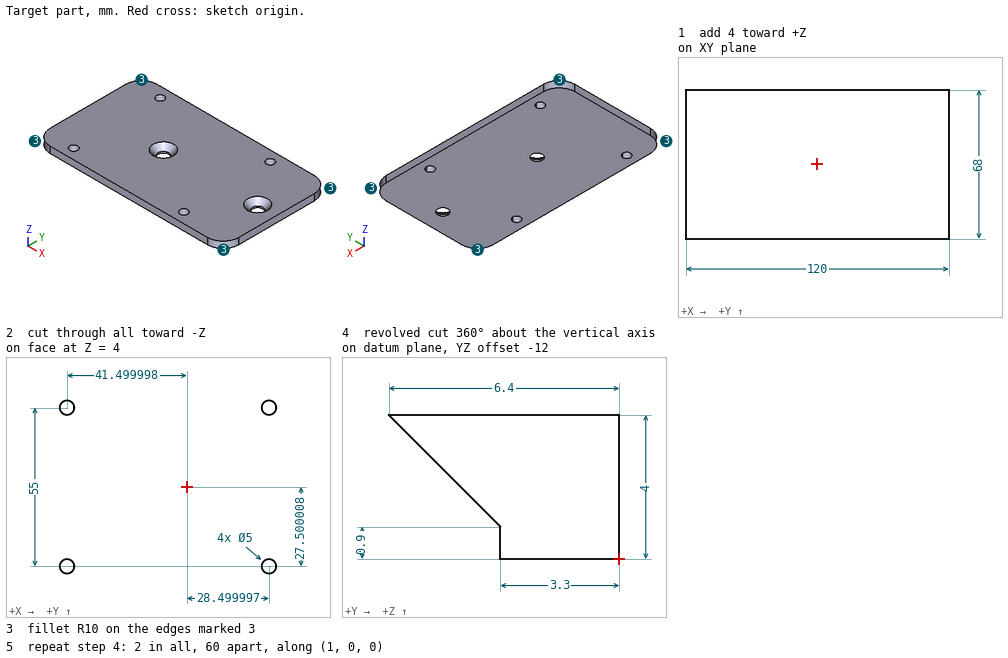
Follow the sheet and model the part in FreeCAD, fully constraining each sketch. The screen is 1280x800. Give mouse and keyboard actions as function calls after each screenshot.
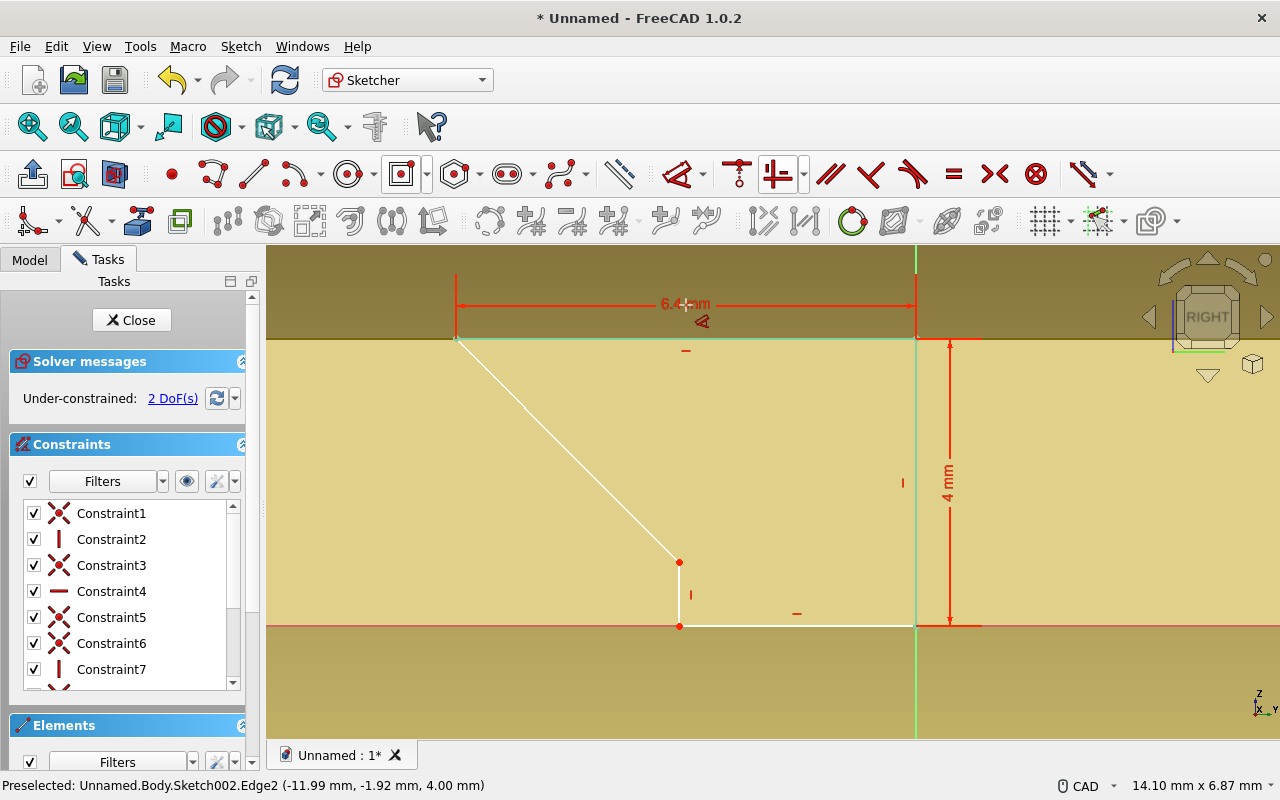
click(679, 582)
click(645, 595)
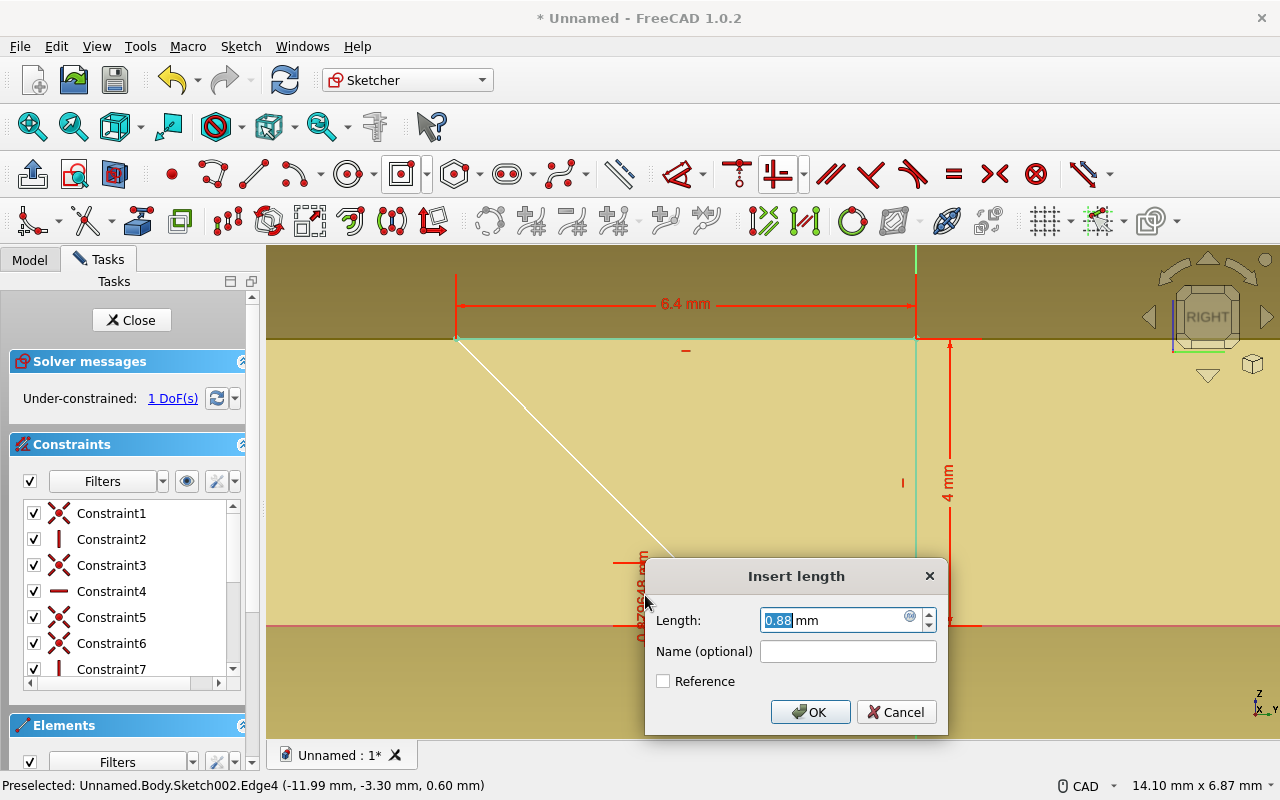
text(0.9)
key(Return)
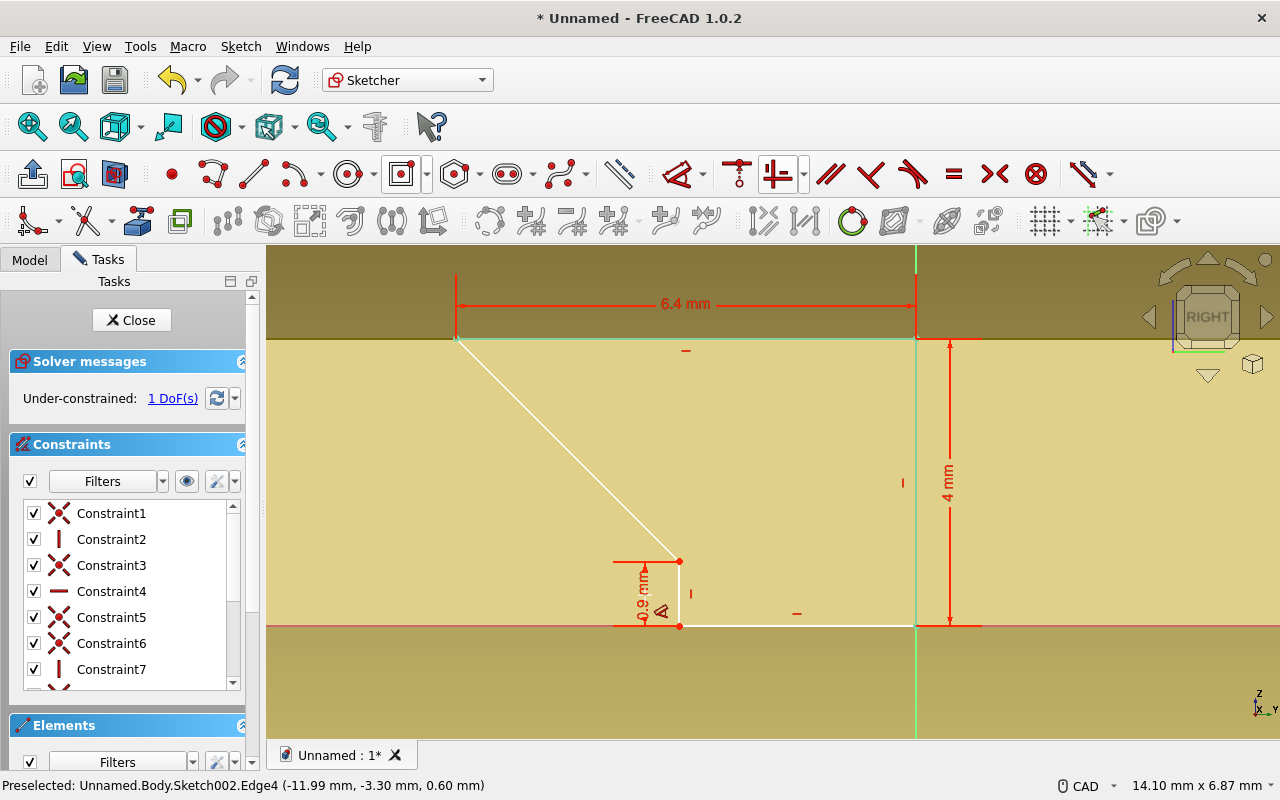
click(750, 626)
click(798, 660)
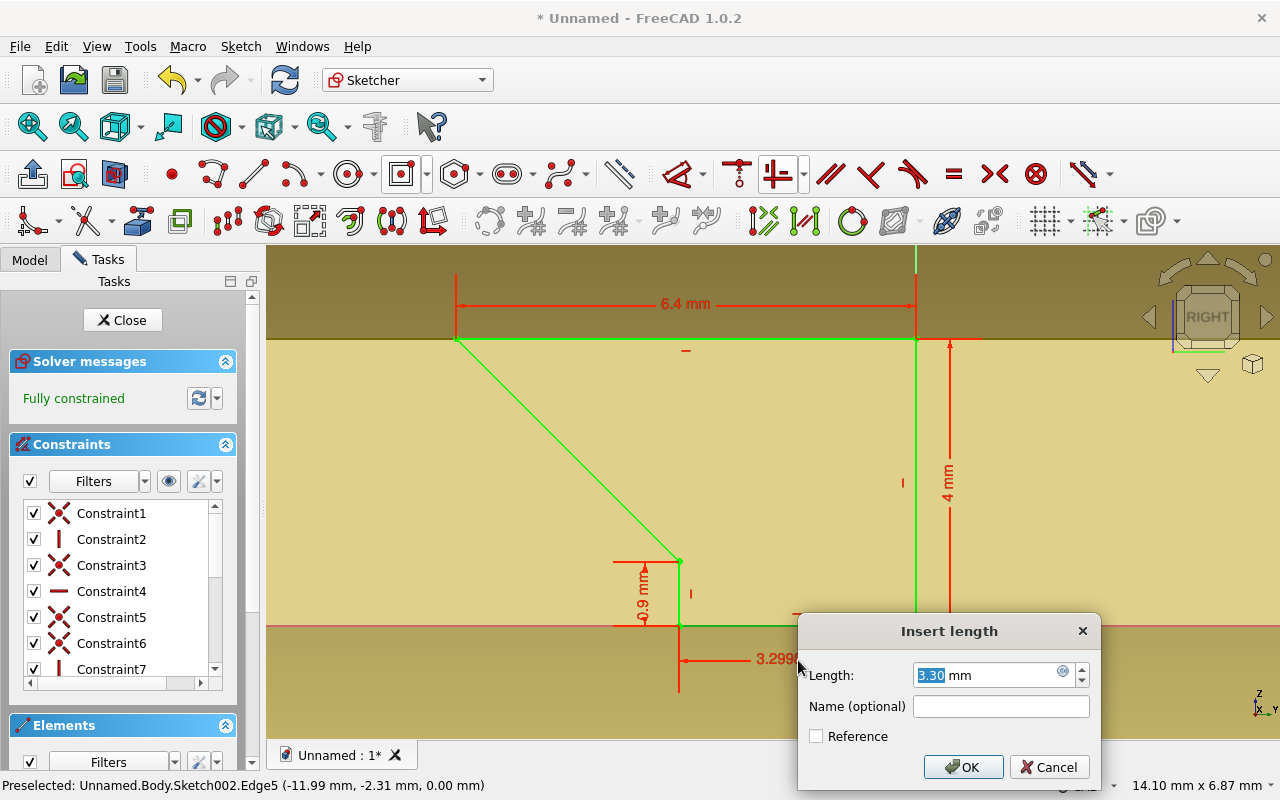
text(3.3)
key(Return)
key(Escape)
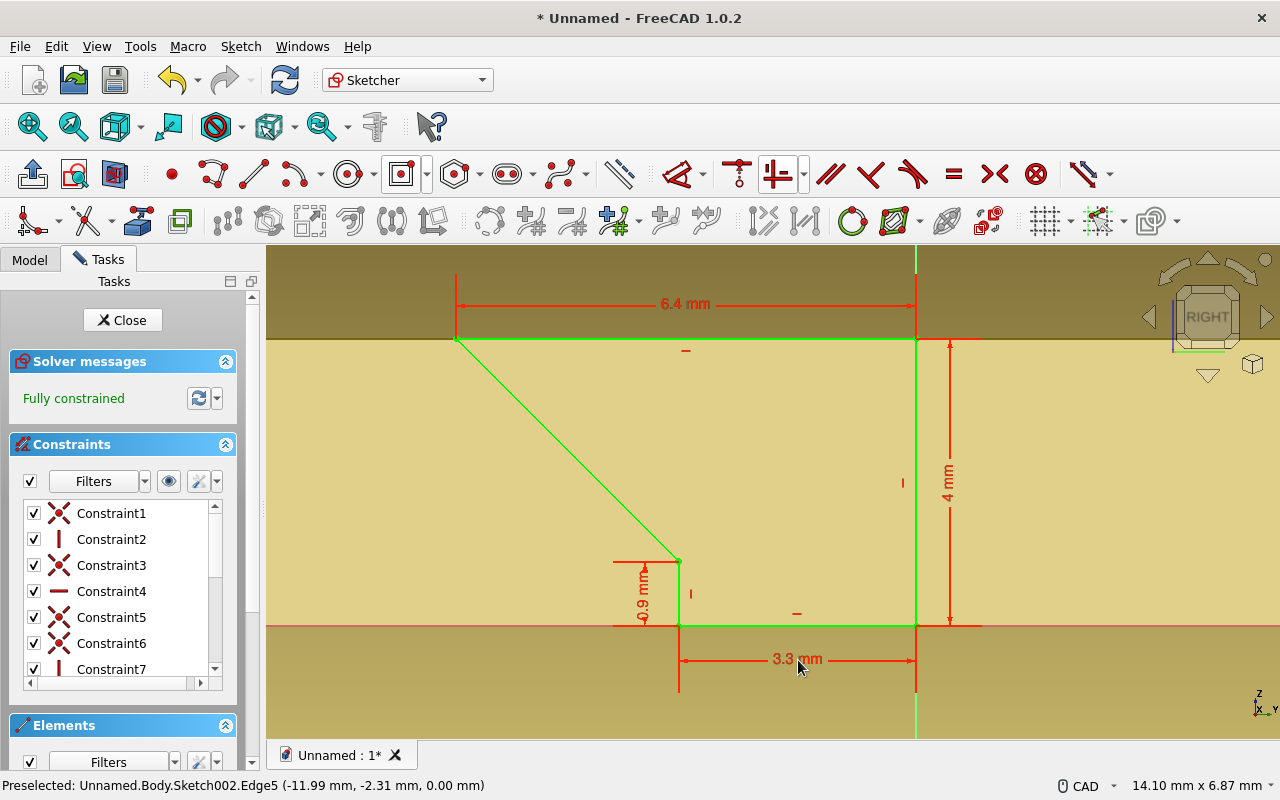
click(123, 320)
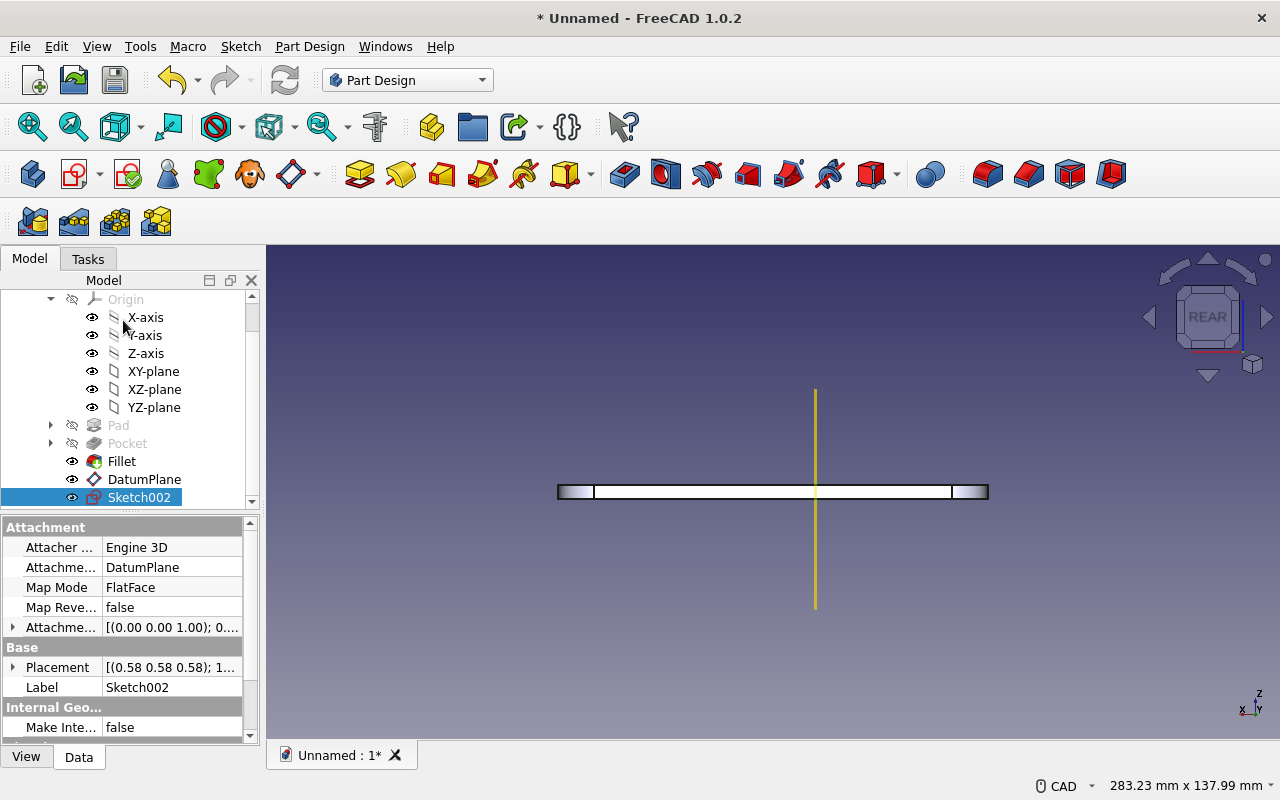
click(707, 174)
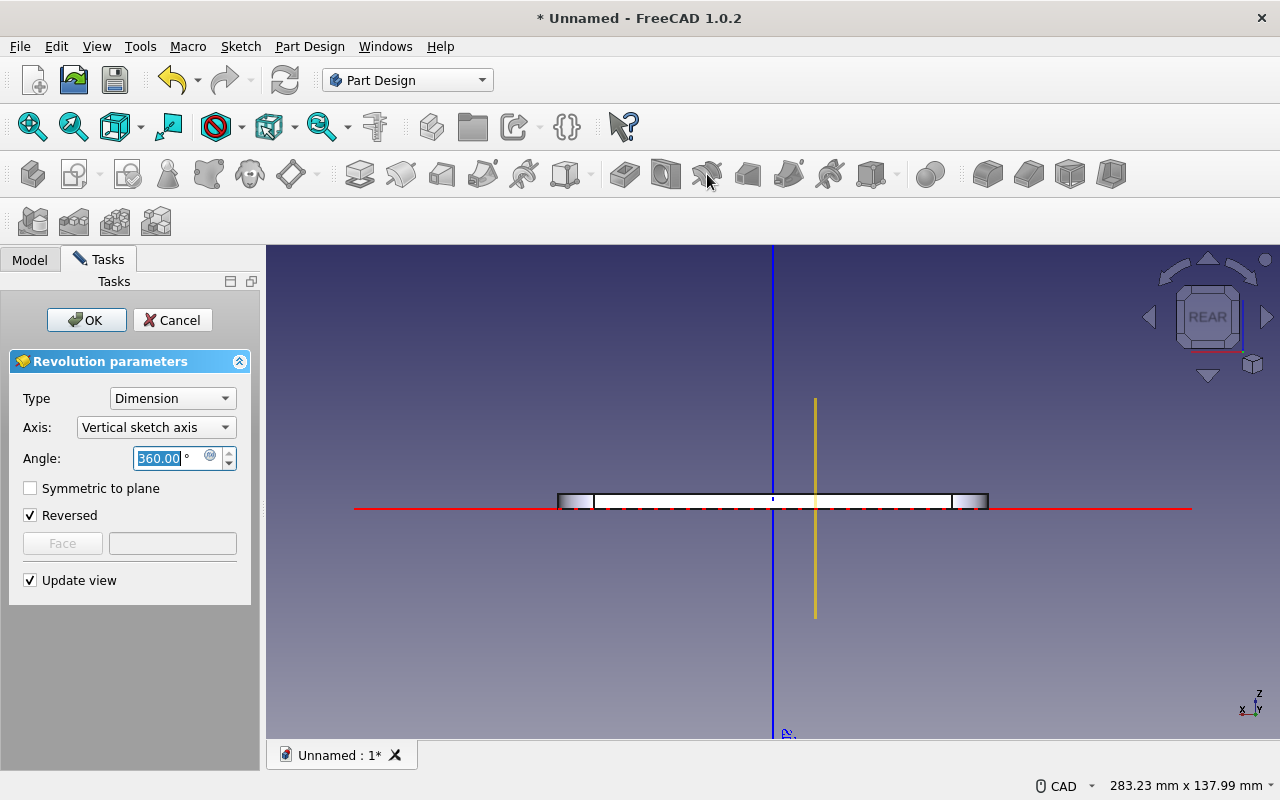
click(87, 320)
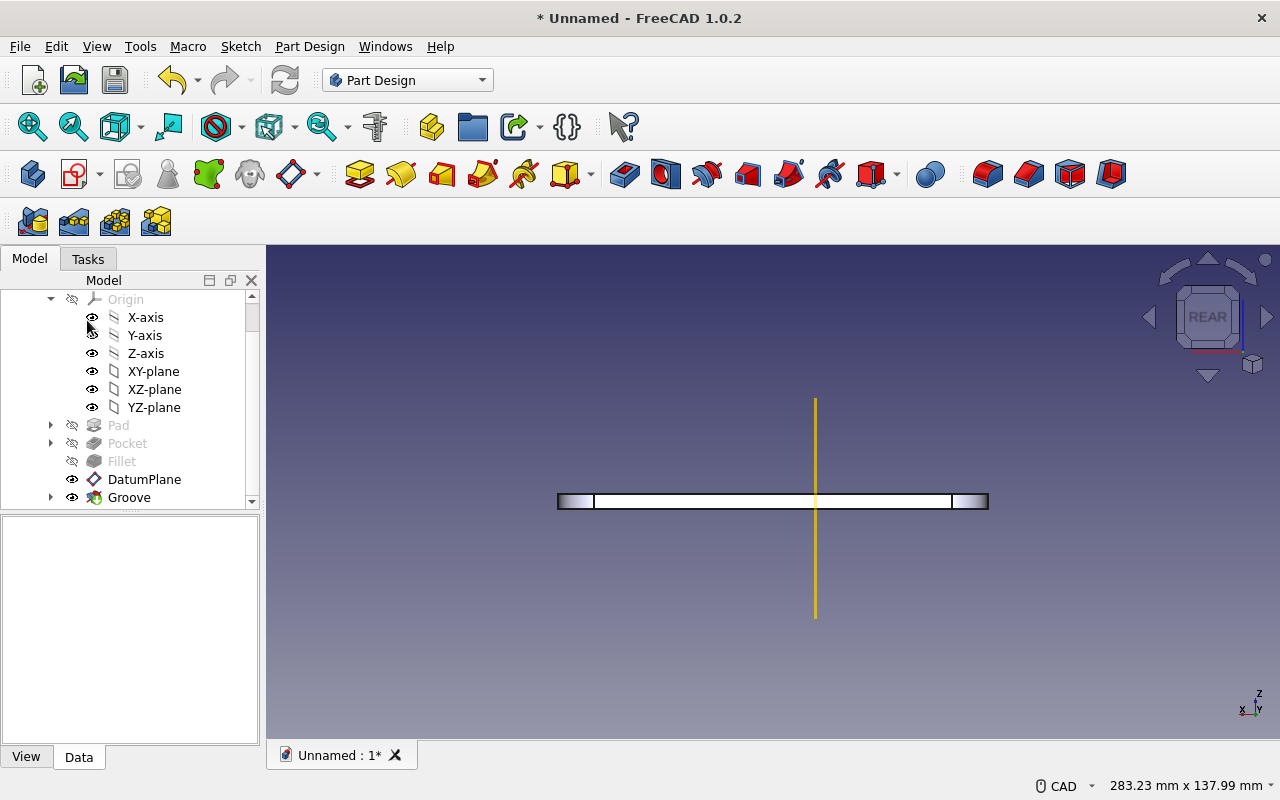
click(117, 479)
key(space)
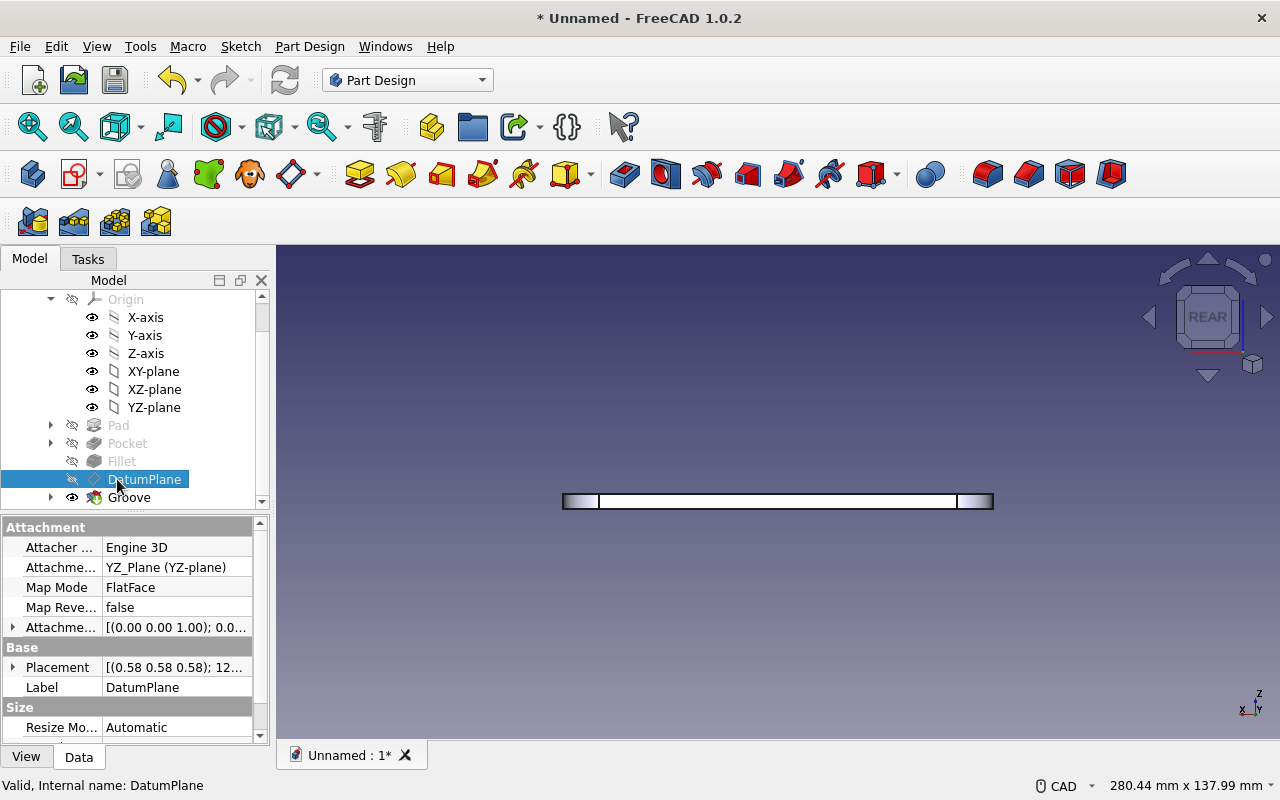
click(33, 128)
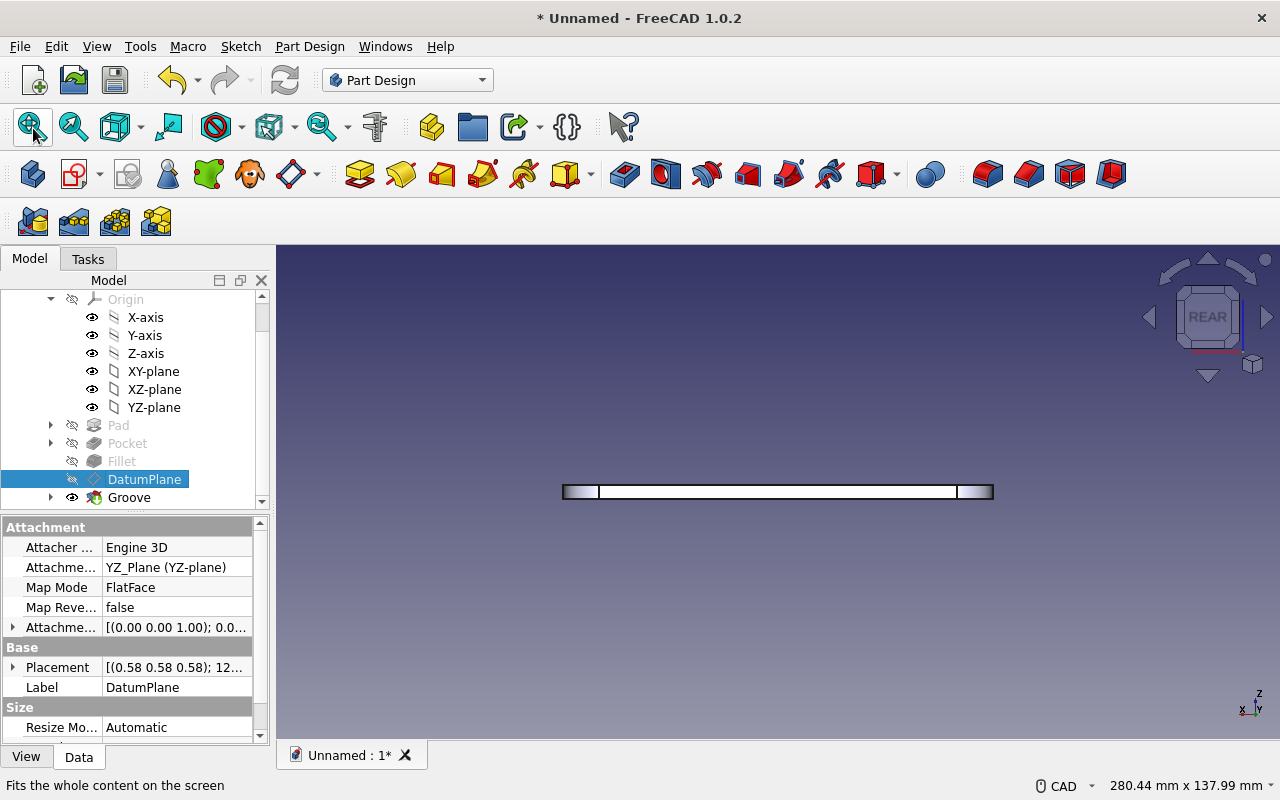
click(117, 497)